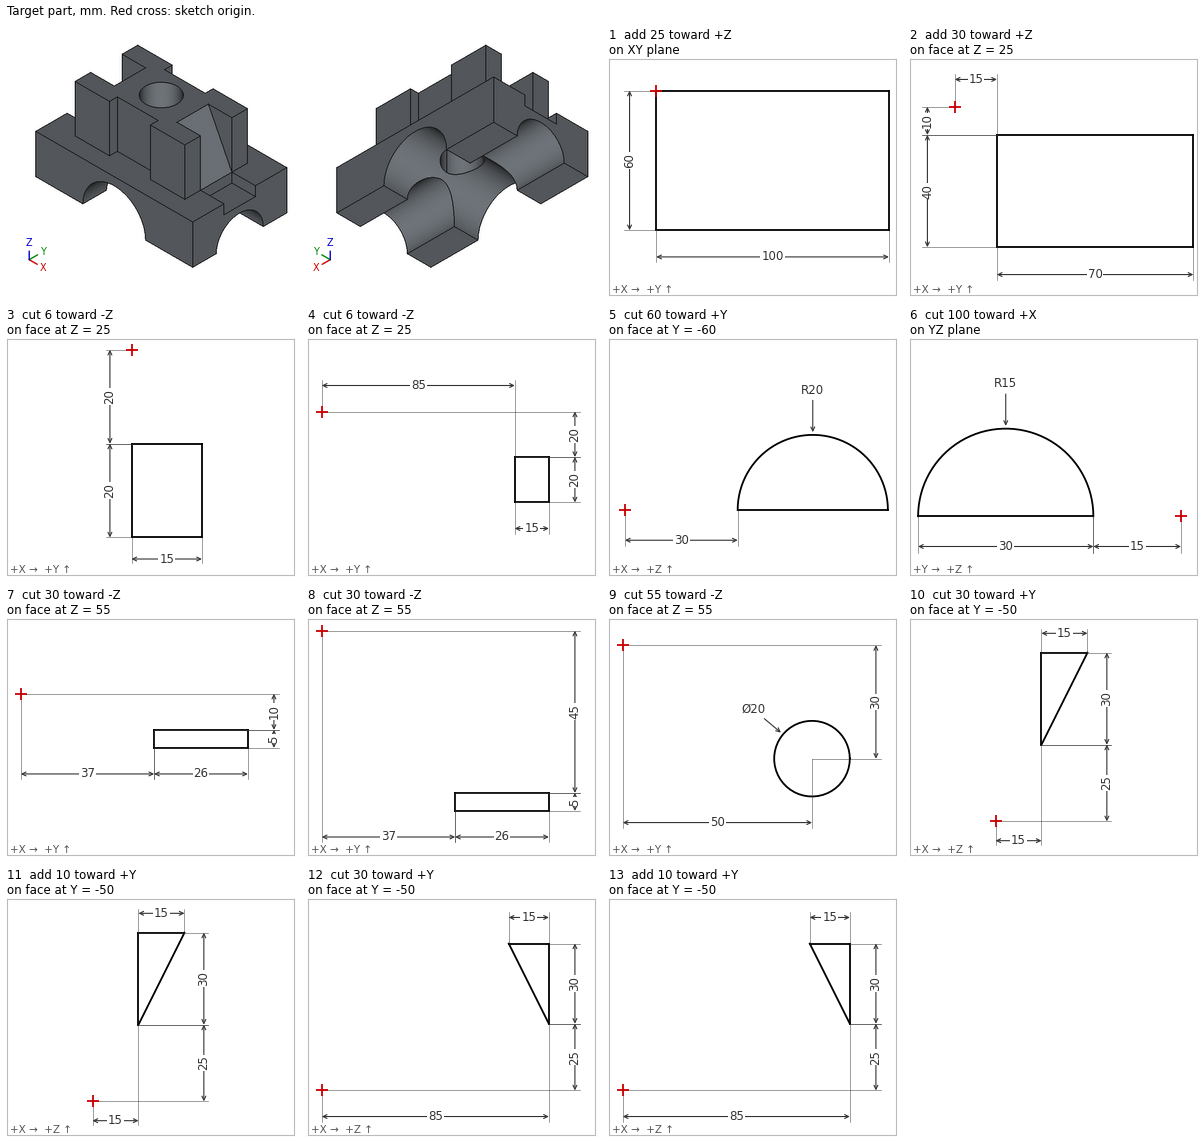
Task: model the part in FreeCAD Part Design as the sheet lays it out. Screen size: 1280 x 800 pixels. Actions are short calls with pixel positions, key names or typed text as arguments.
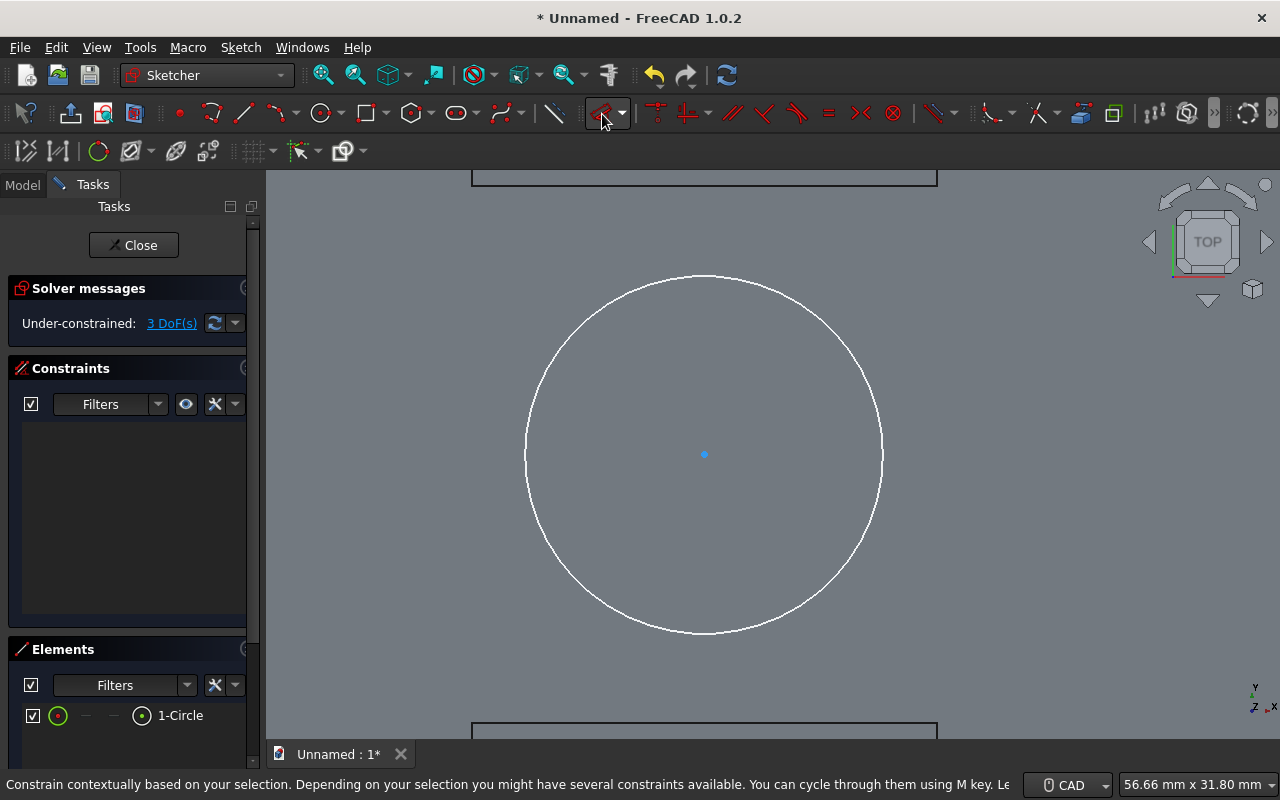
click(830, 328)
click(853, 305)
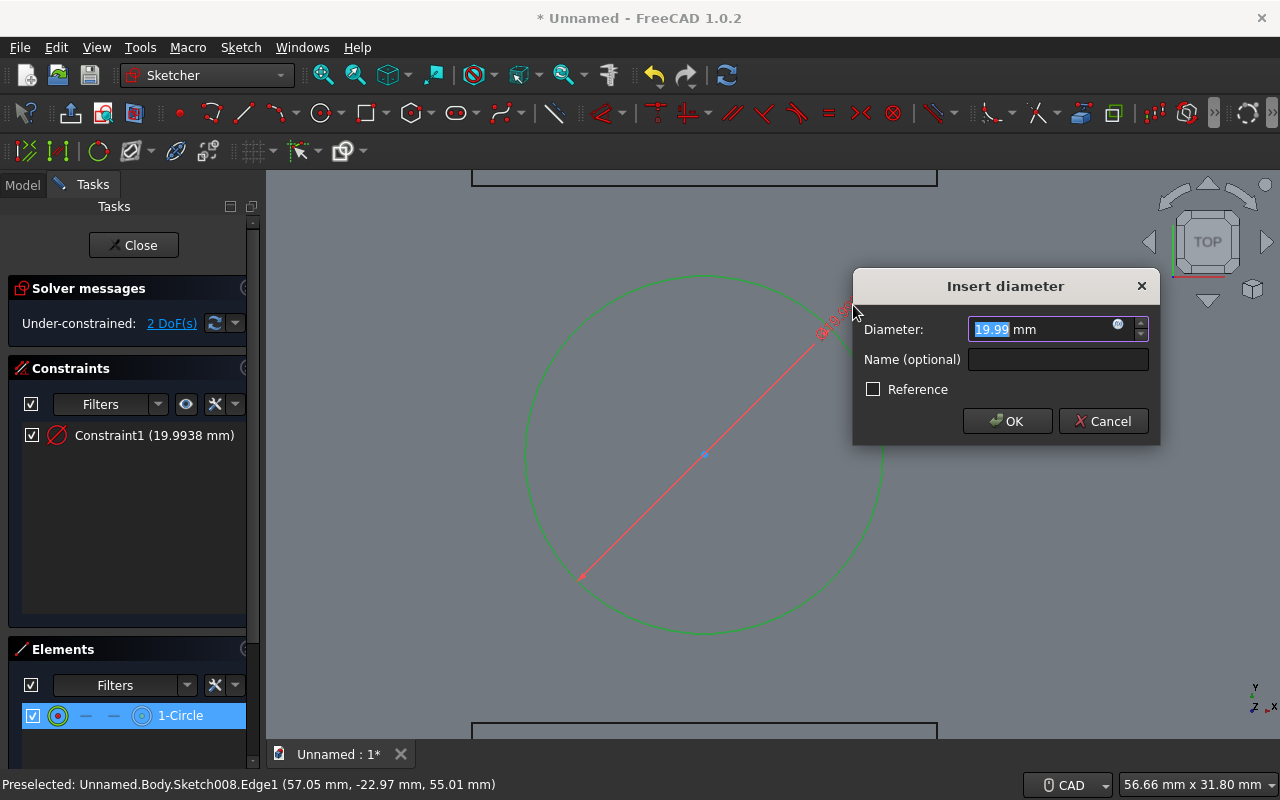
text(20)
key(Return)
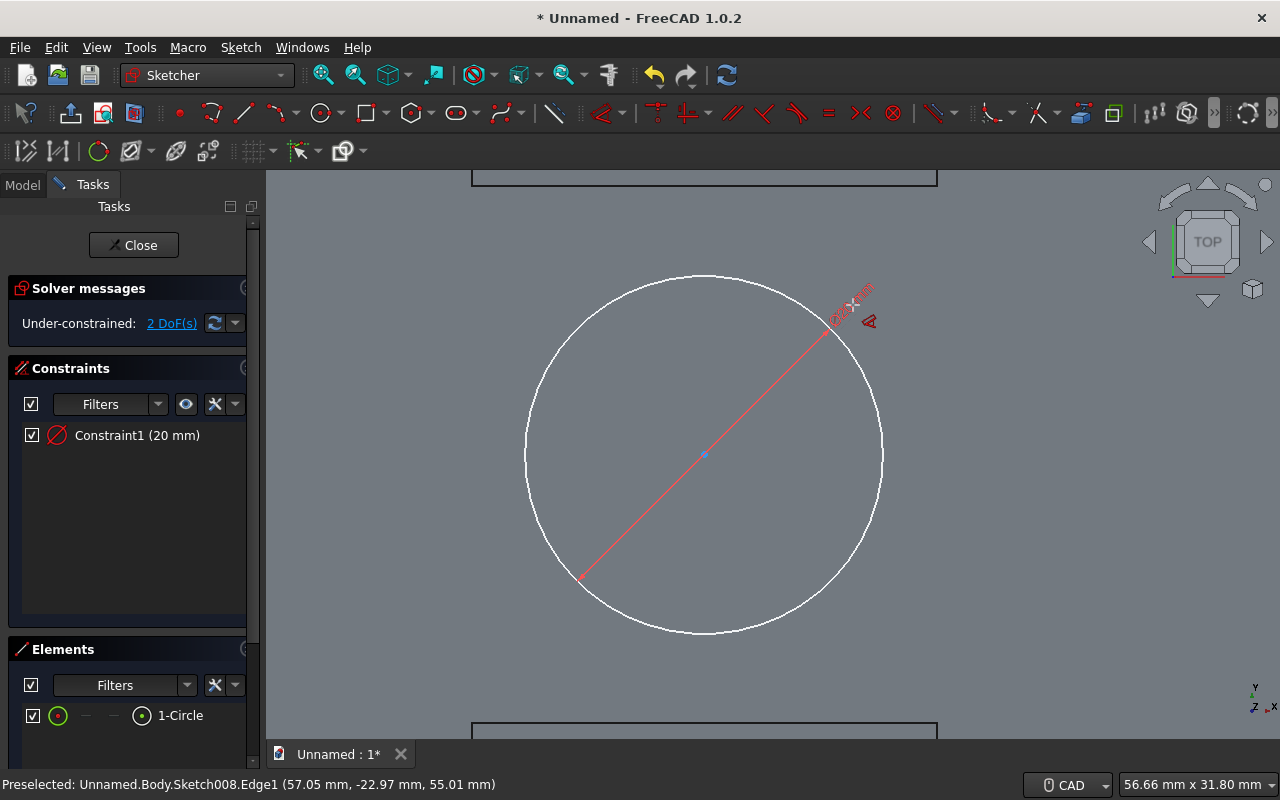
click(704, 455)
click(499, 489)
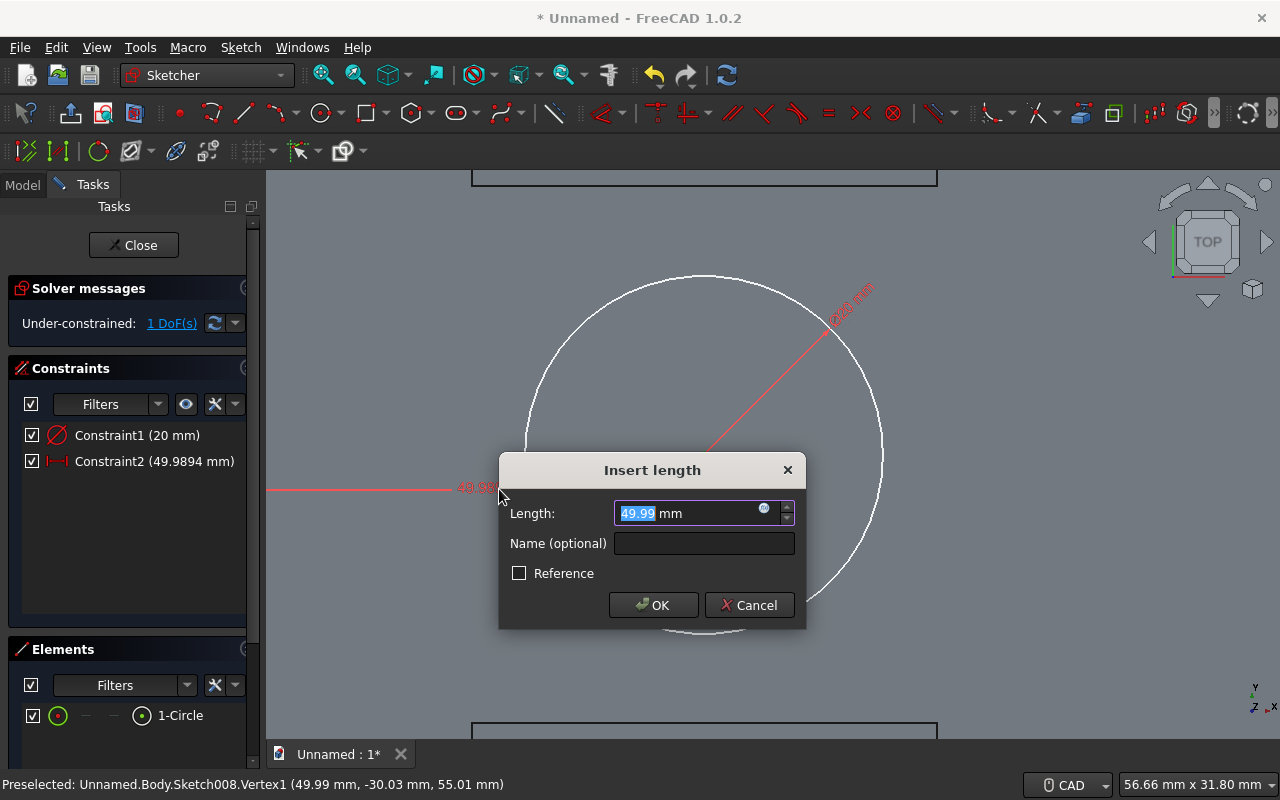
text(50)
key(Return)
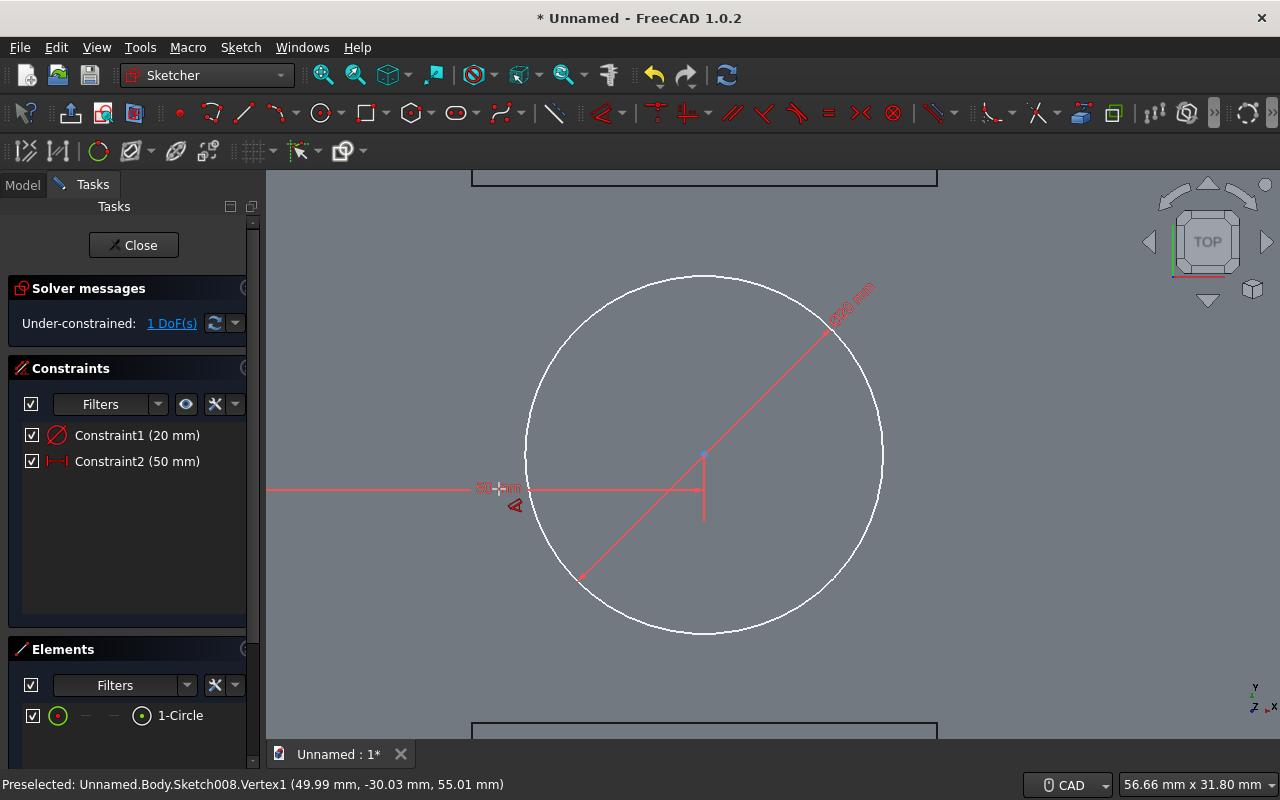
click(704, 455)
click(738, 326)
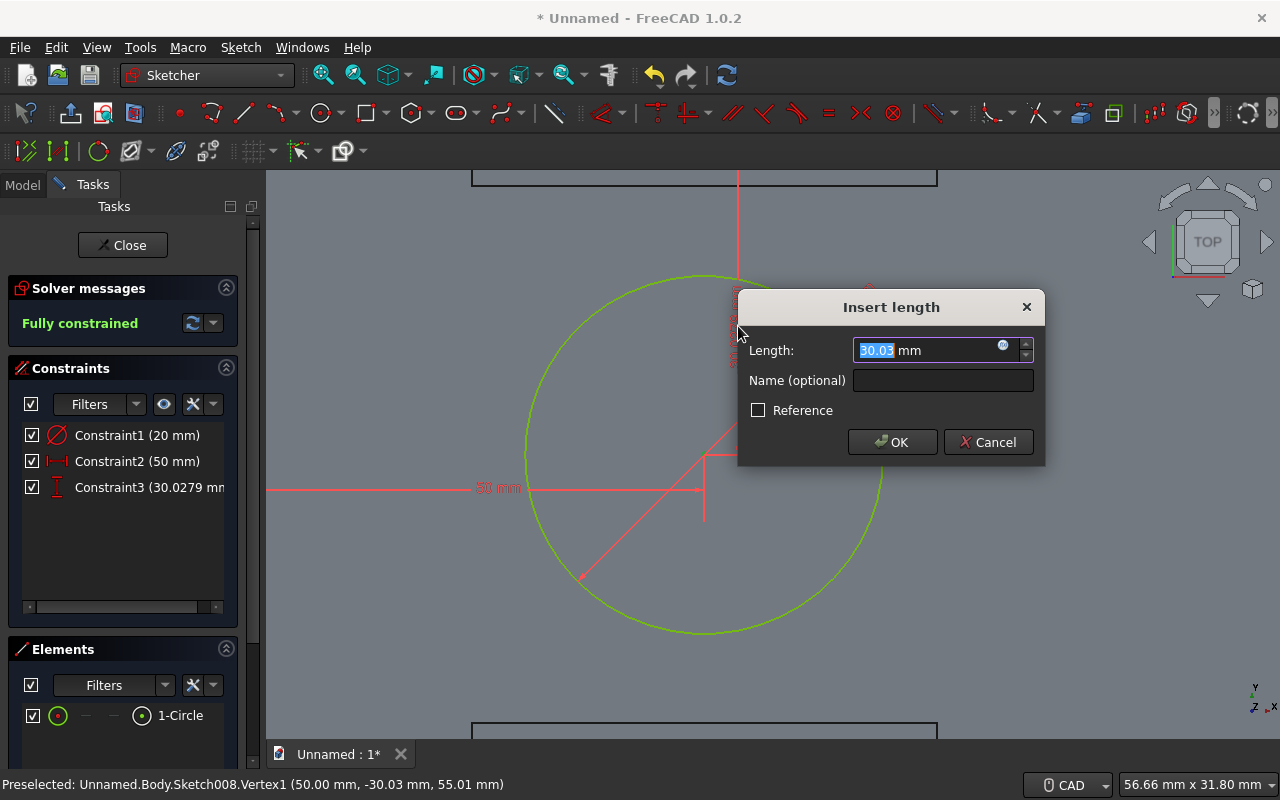
text(30)
key(Return)
key(Escape)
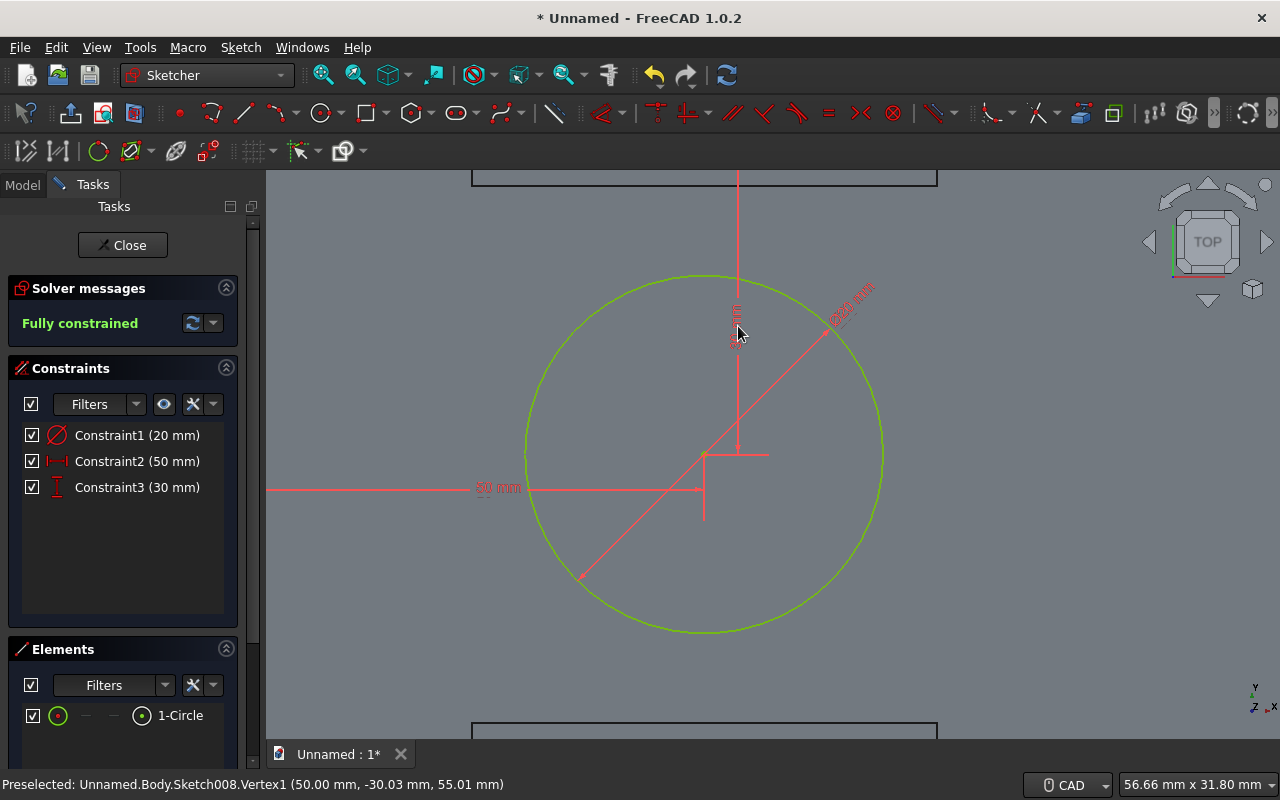
click(123, 245)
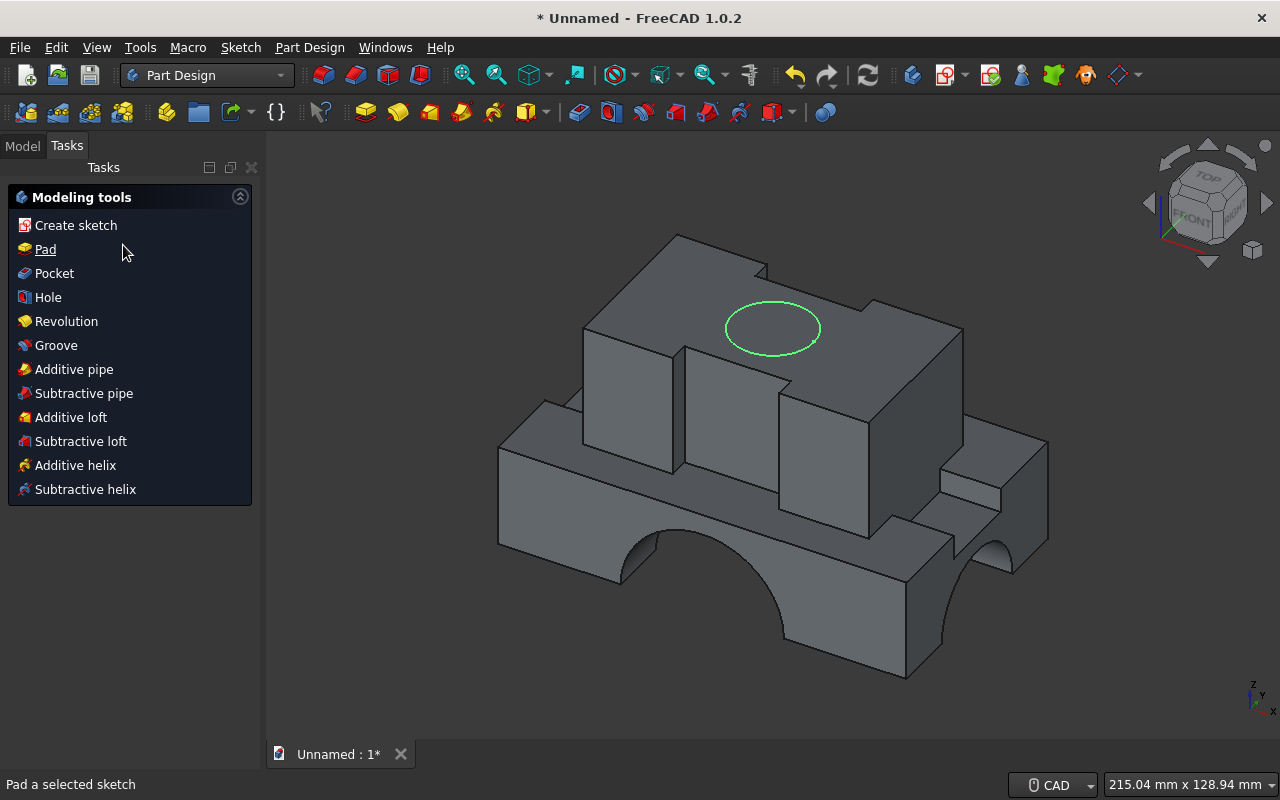
click(580, 112)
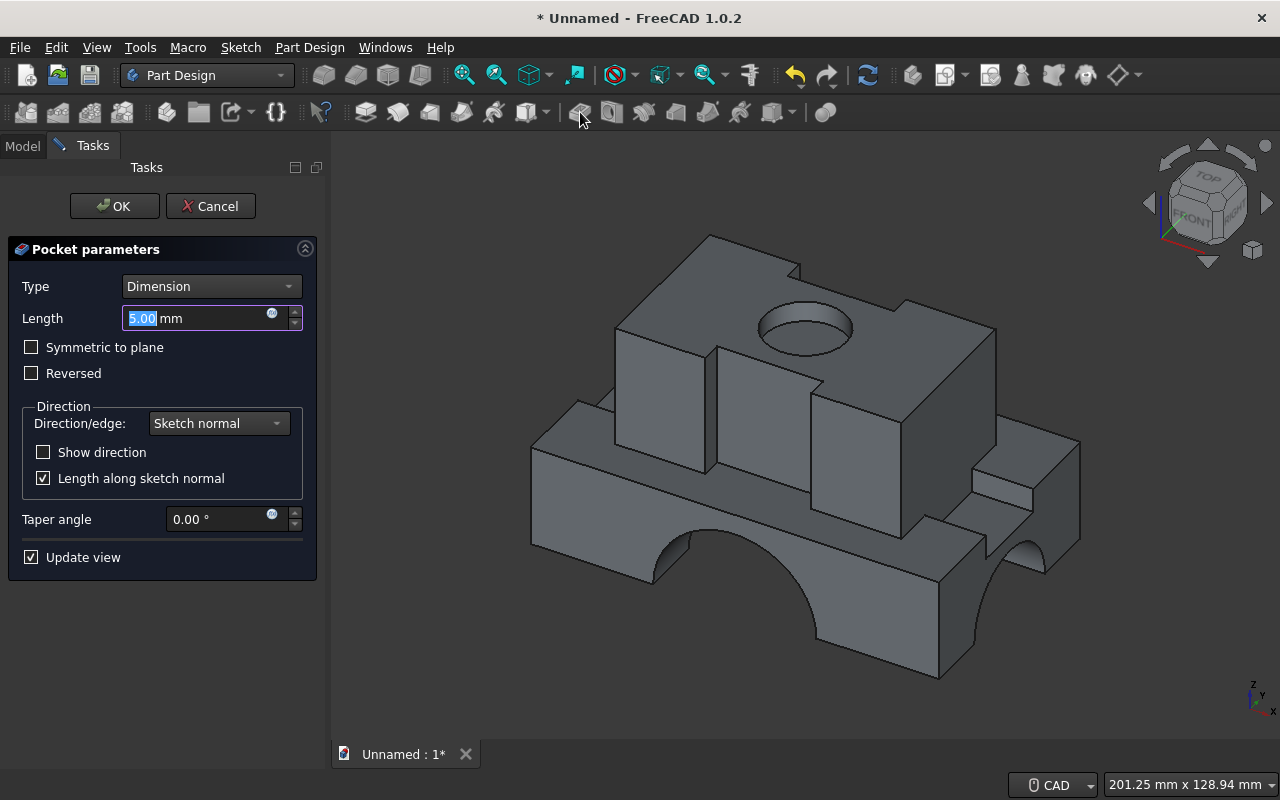
text(55)
key(Tab)